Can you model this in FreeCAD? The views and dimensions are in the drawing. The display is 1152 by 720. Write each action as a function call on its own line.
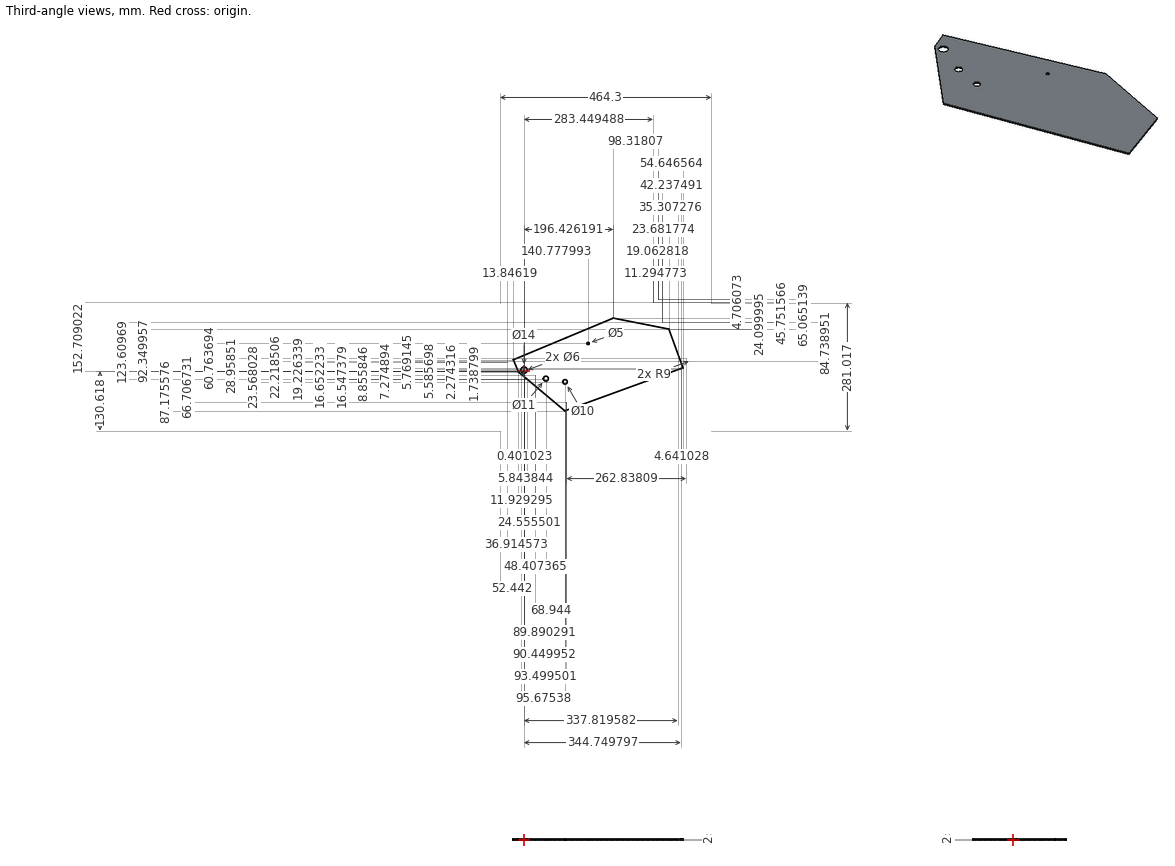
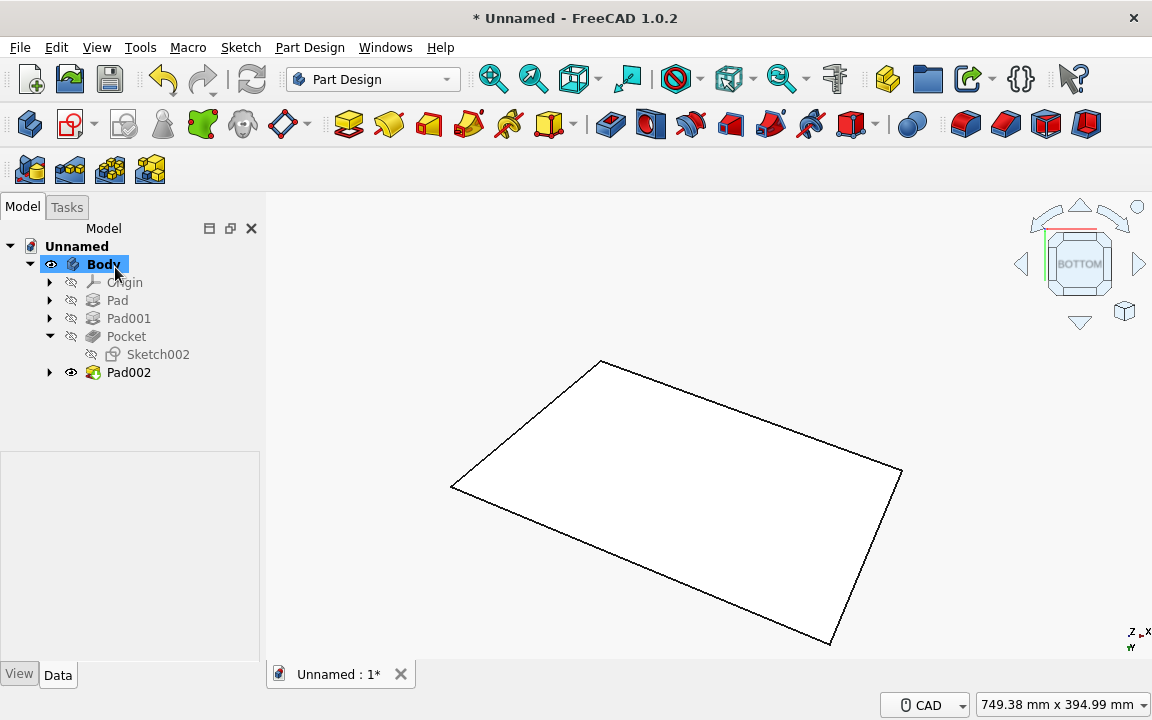
click(741, 502)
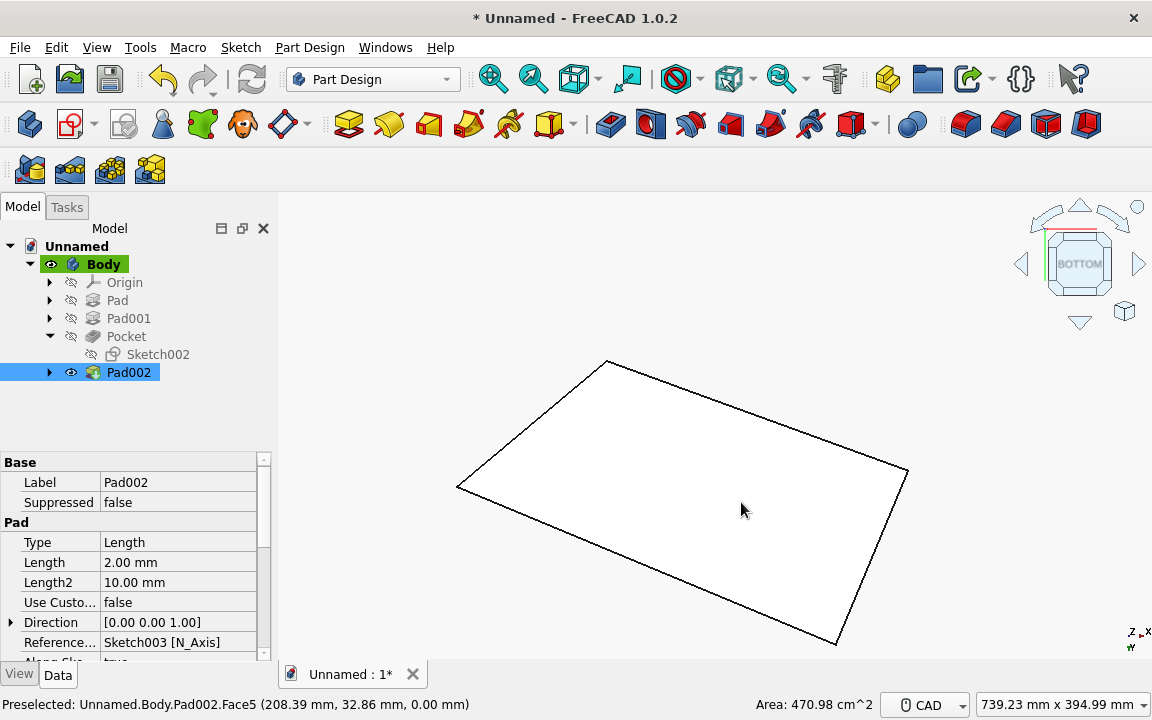
click(70, 124)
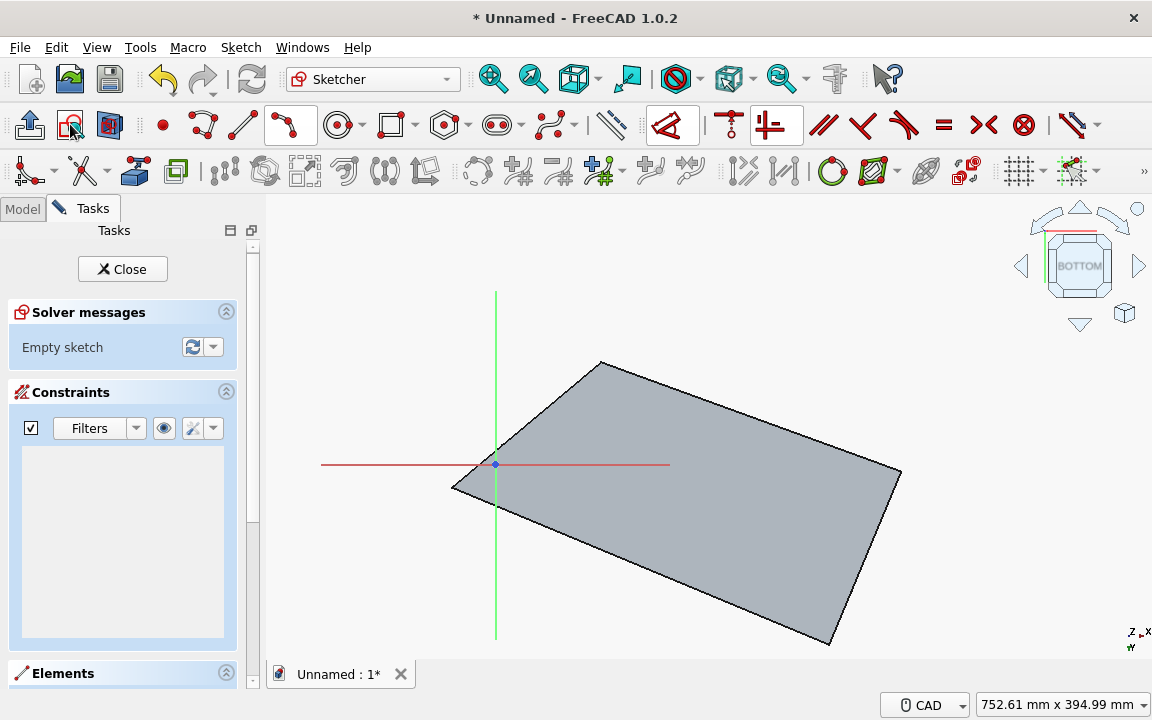
scroll(487, 470, up, 14)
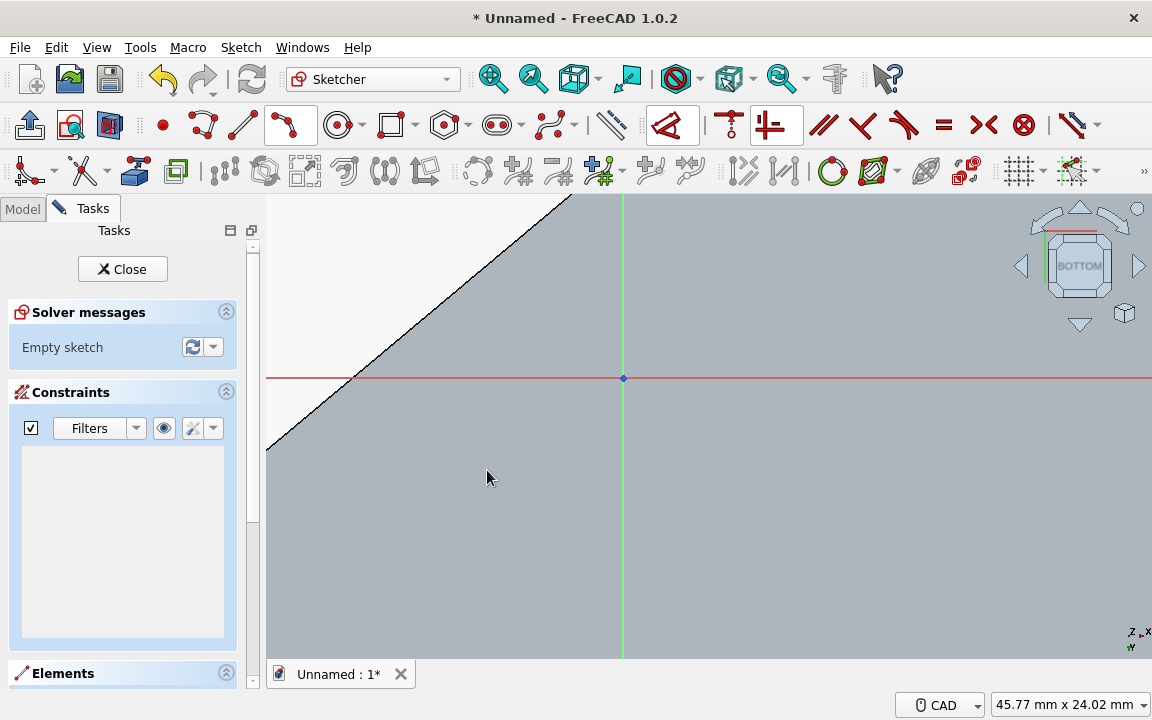
click(338, 126)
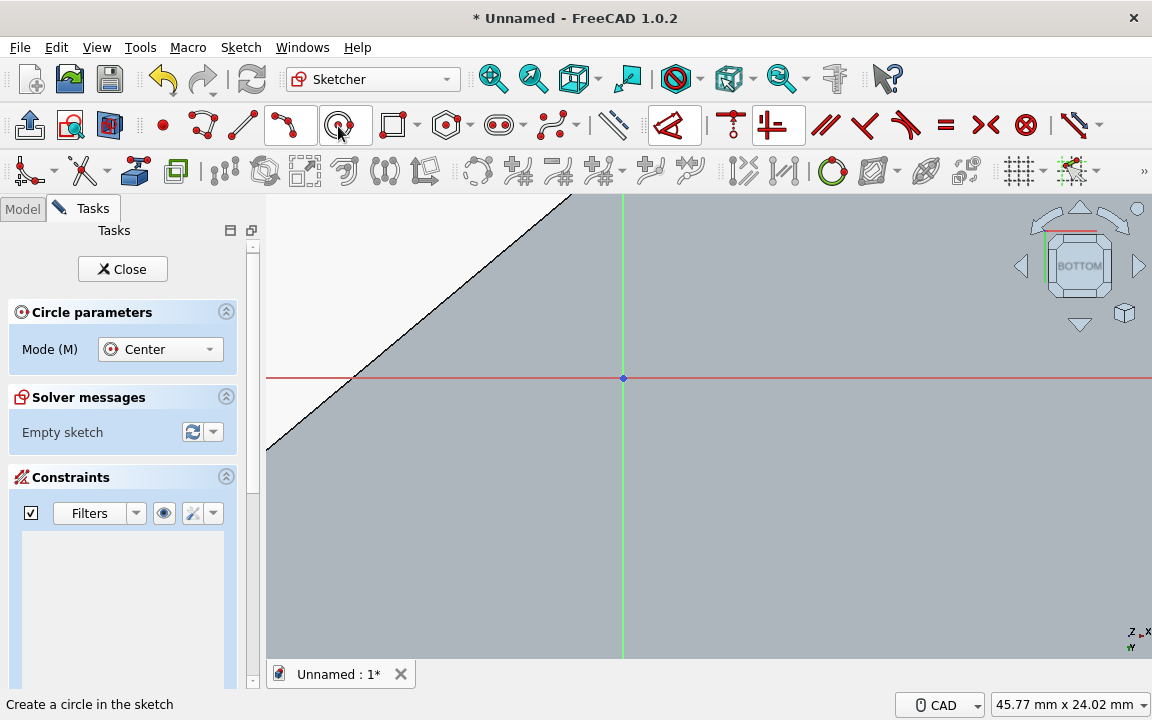
scroll(631, 422, up, 4)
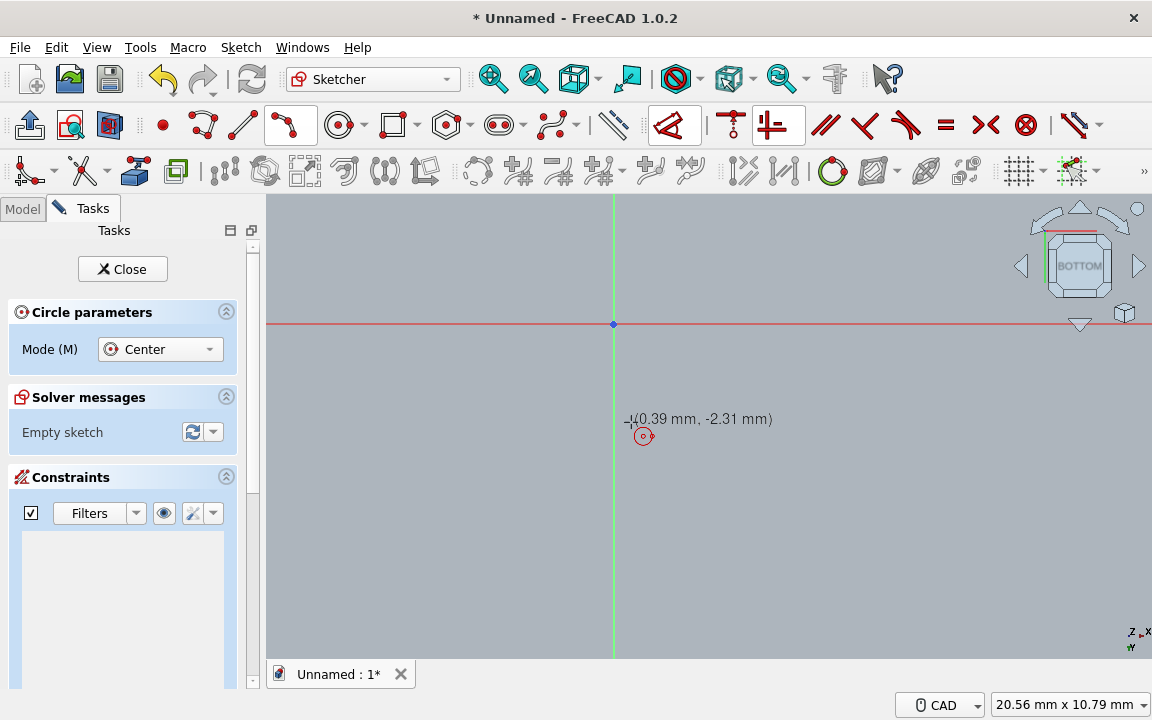
click(631, 422)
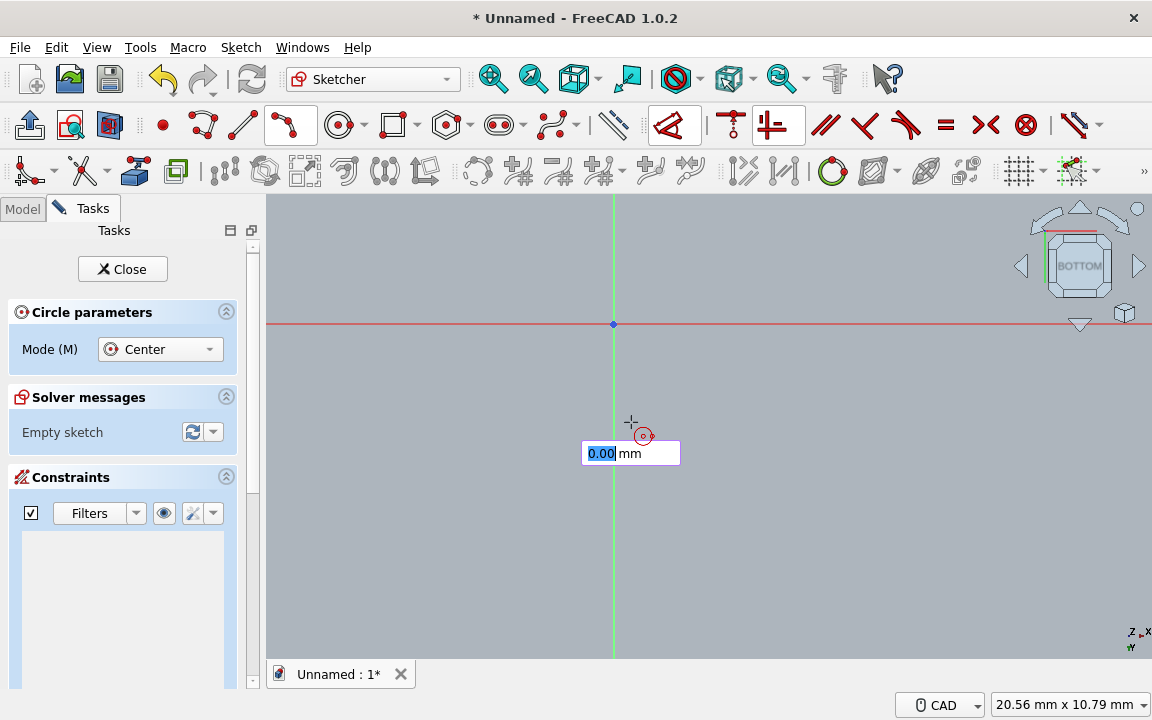
scroll(648, 430, down, 4)
move(736, 331)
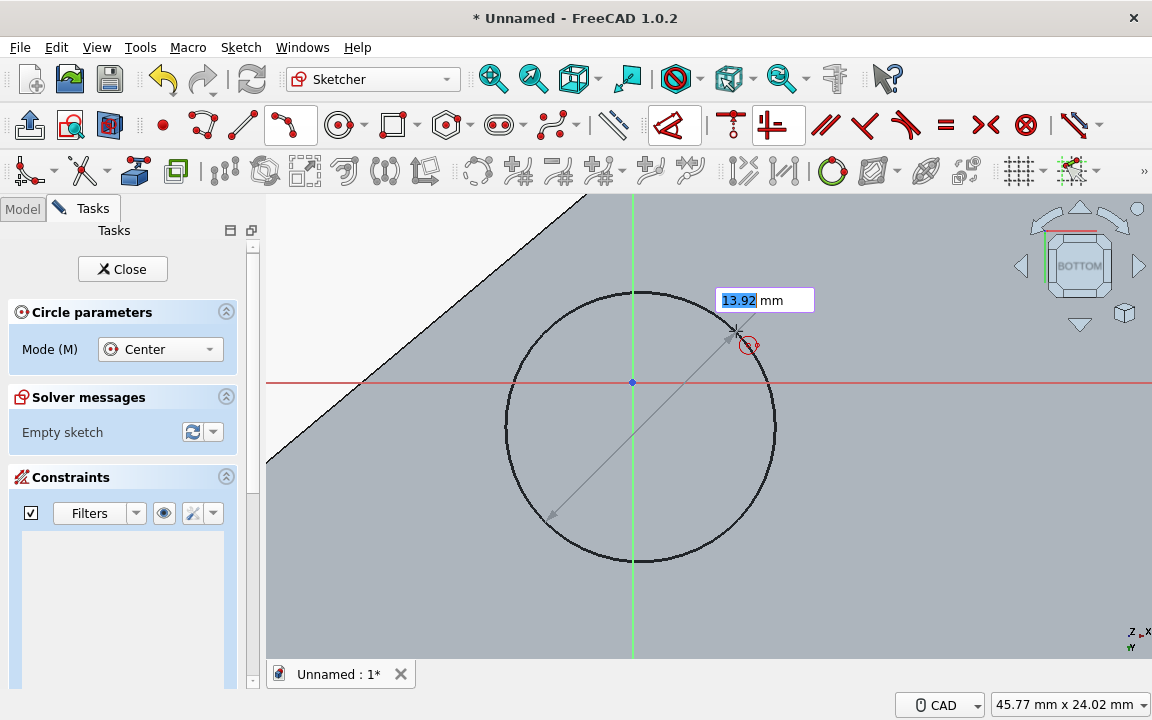
text(14)
key(Return)
key(Escape)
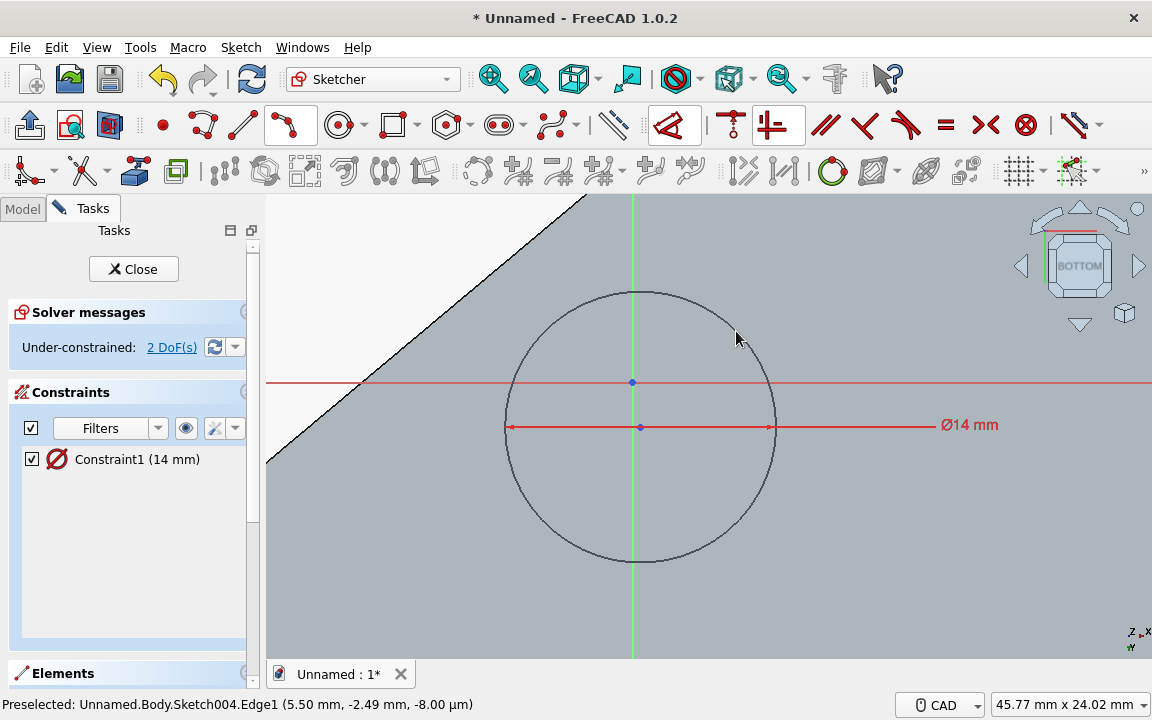
scroll(641, 427, up, 9)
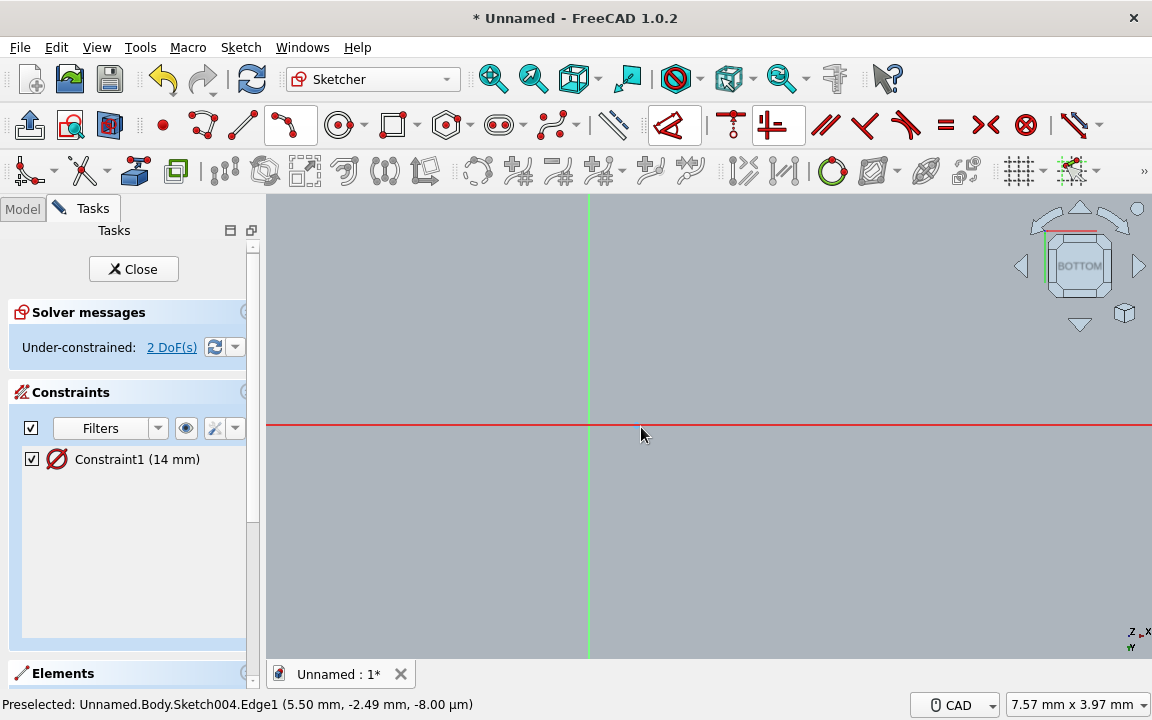
click(636, 425)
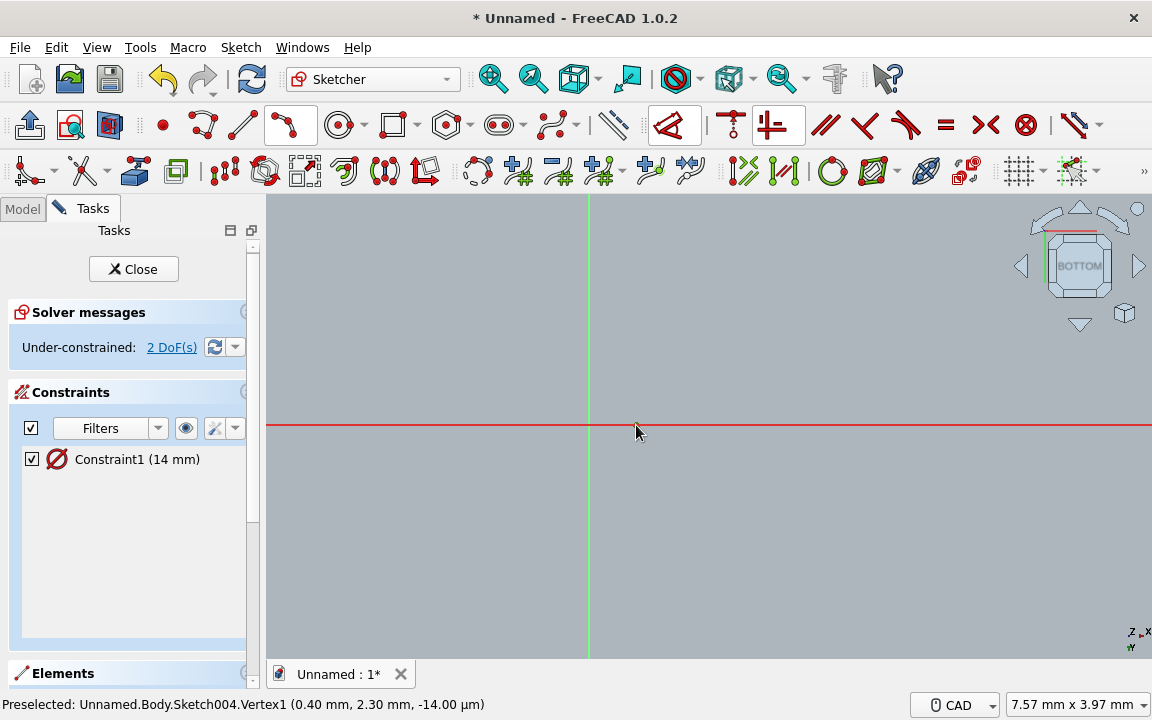
key(l)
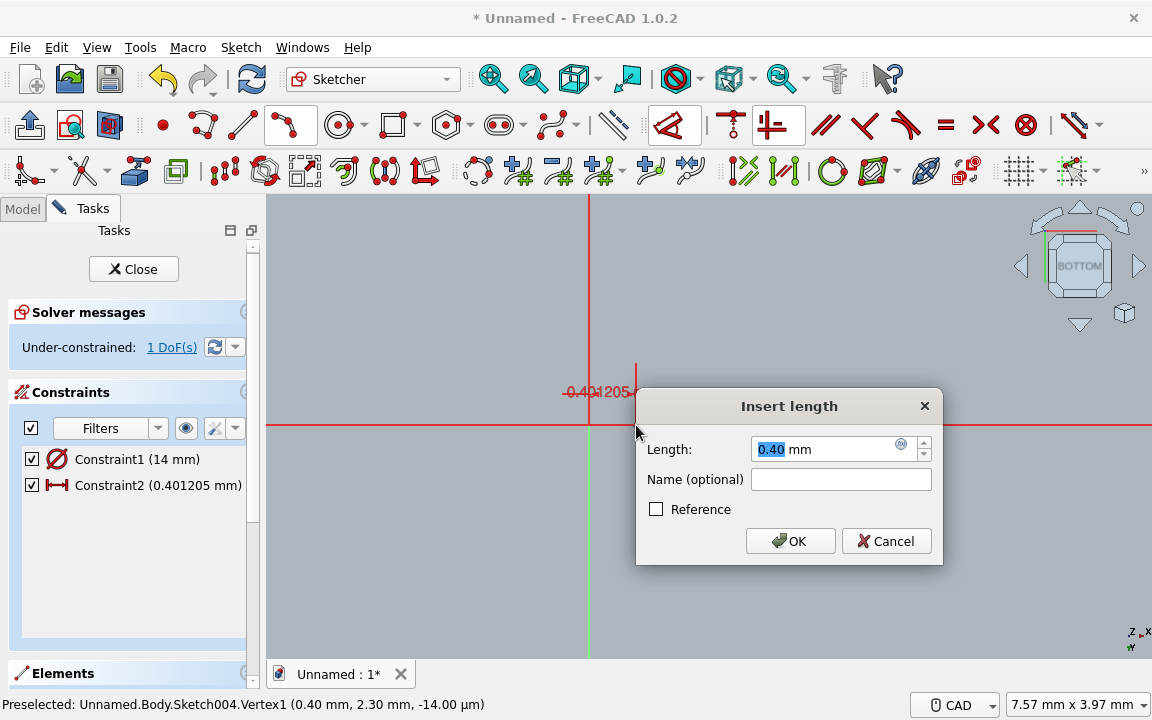
text(0.401023)
key(Return)